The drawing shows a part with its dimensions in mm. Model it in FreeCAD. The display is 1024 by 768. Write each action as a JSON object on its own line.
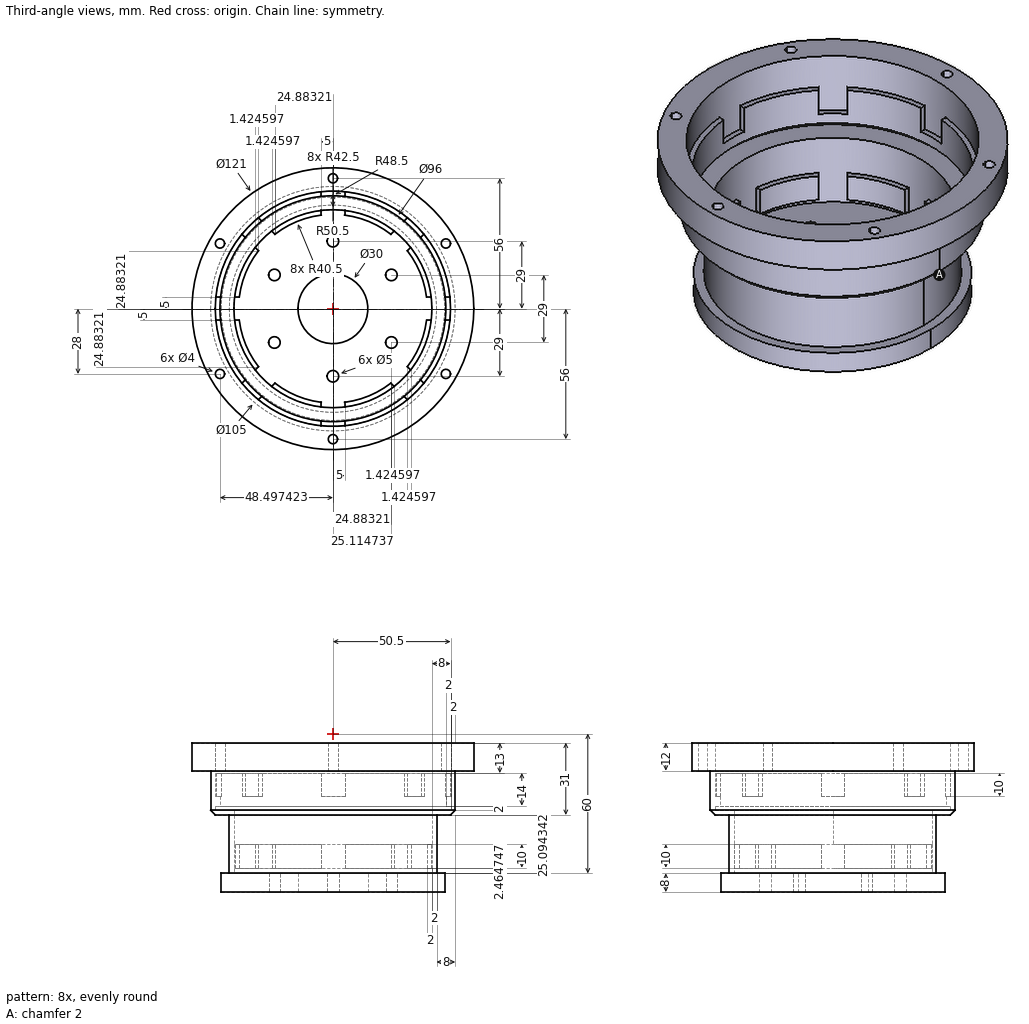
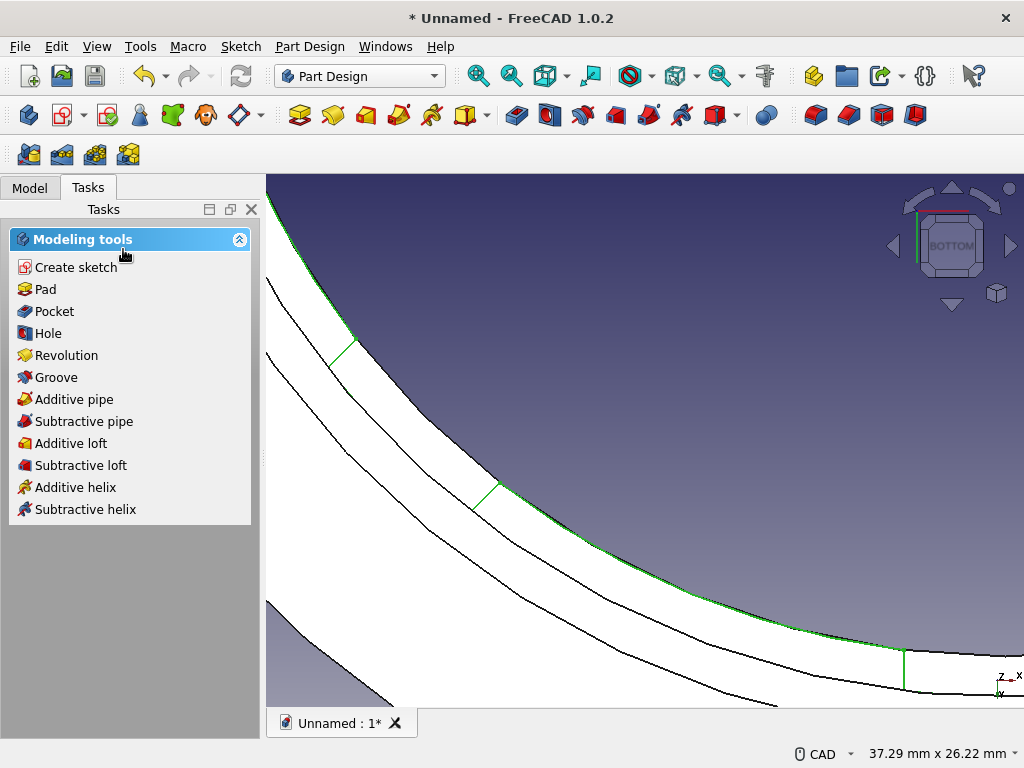
{"action": "left_click", "coordinate": [517, 116]}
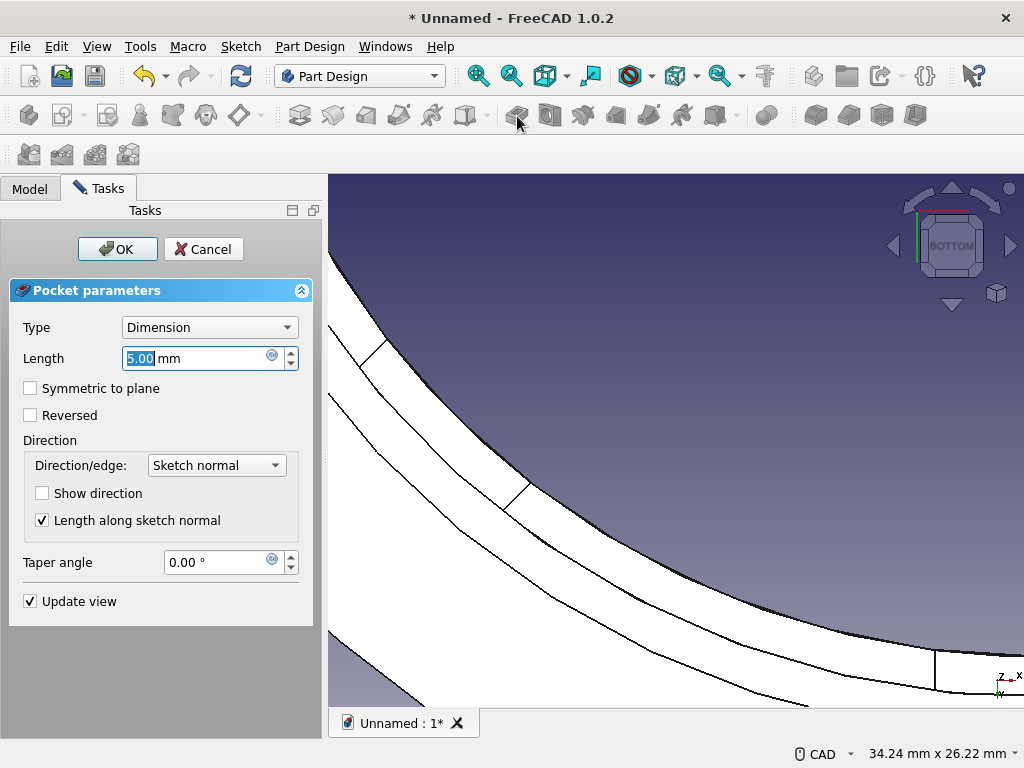
{"action": "type", "text": "10"}
{"action": "key", "text": "Tab"}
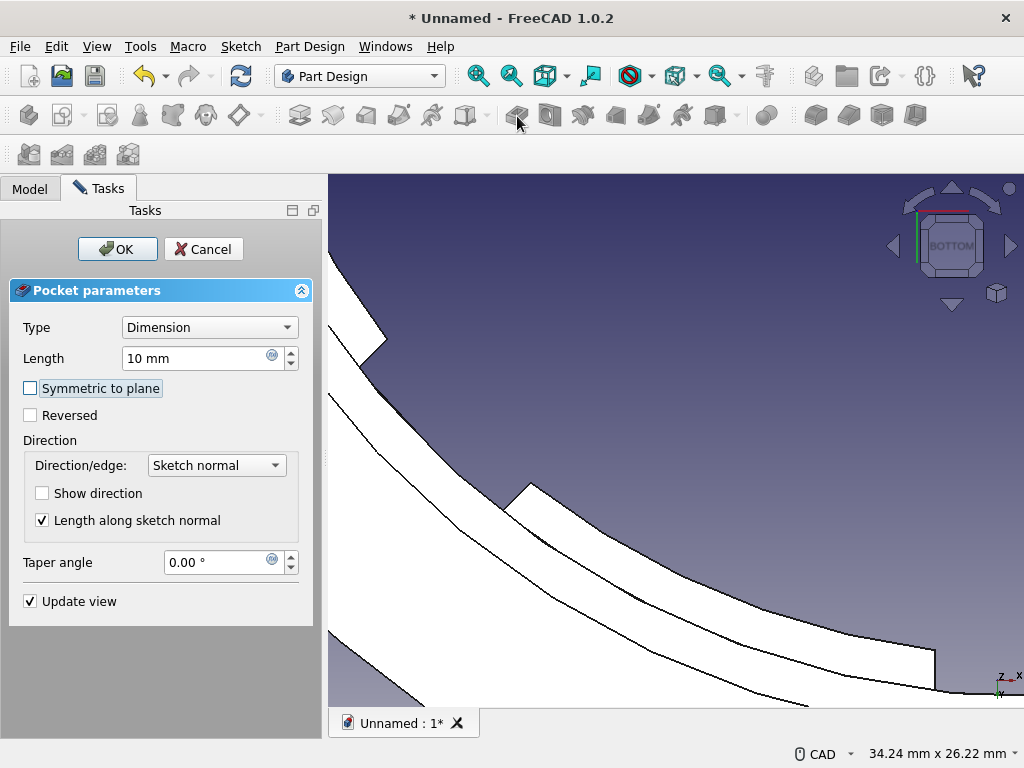
{"action": "left_click", "coordinate": [118, 249]}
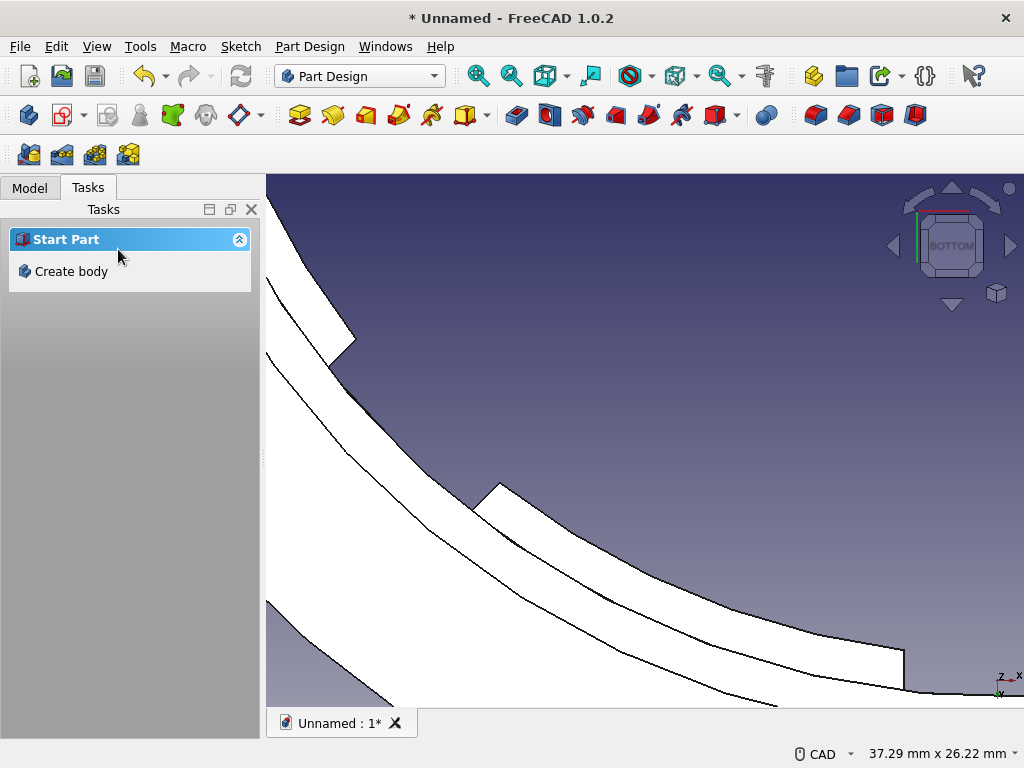
{"action": "left_click", "coordinate": [479, 76]}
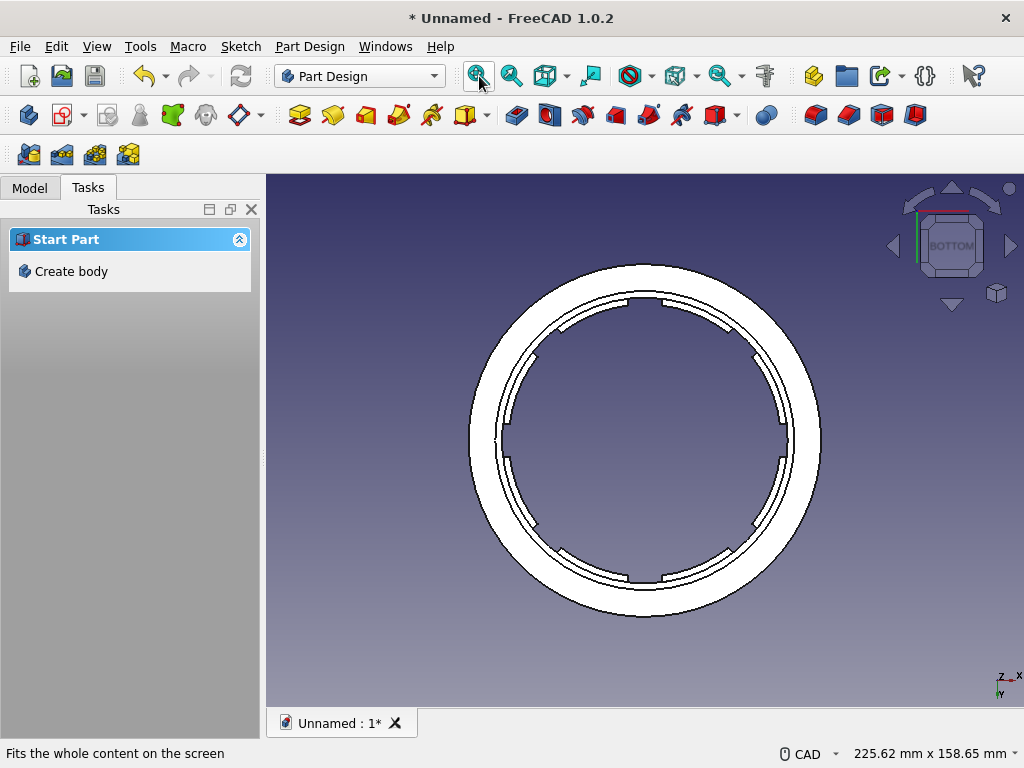
{"action": "left_click", "coordinate": [30, 188]}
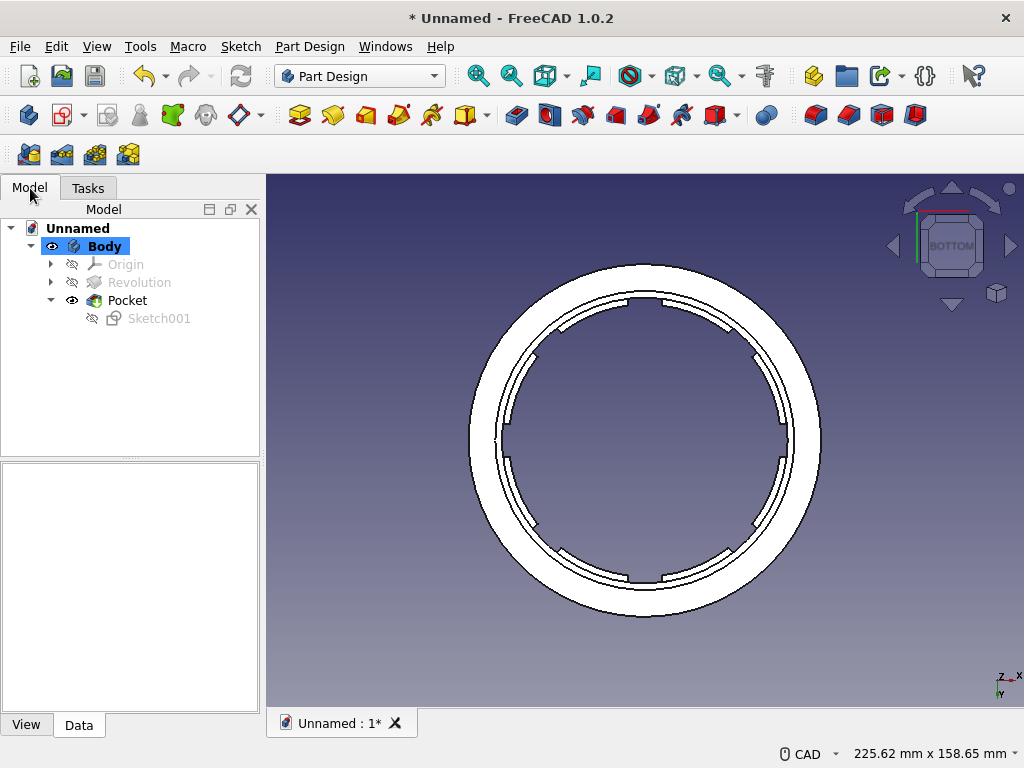
{"action": "left_click", "coordinate": [51, 264]}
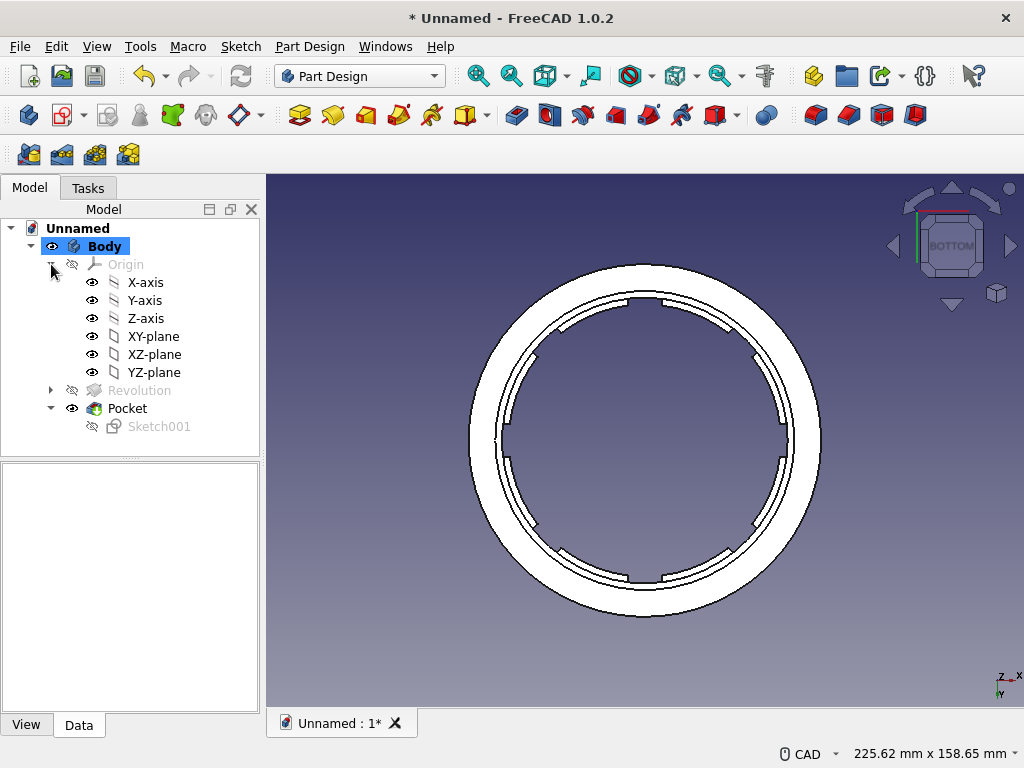
{"action": "left_click", "coordinate": [137, 336]}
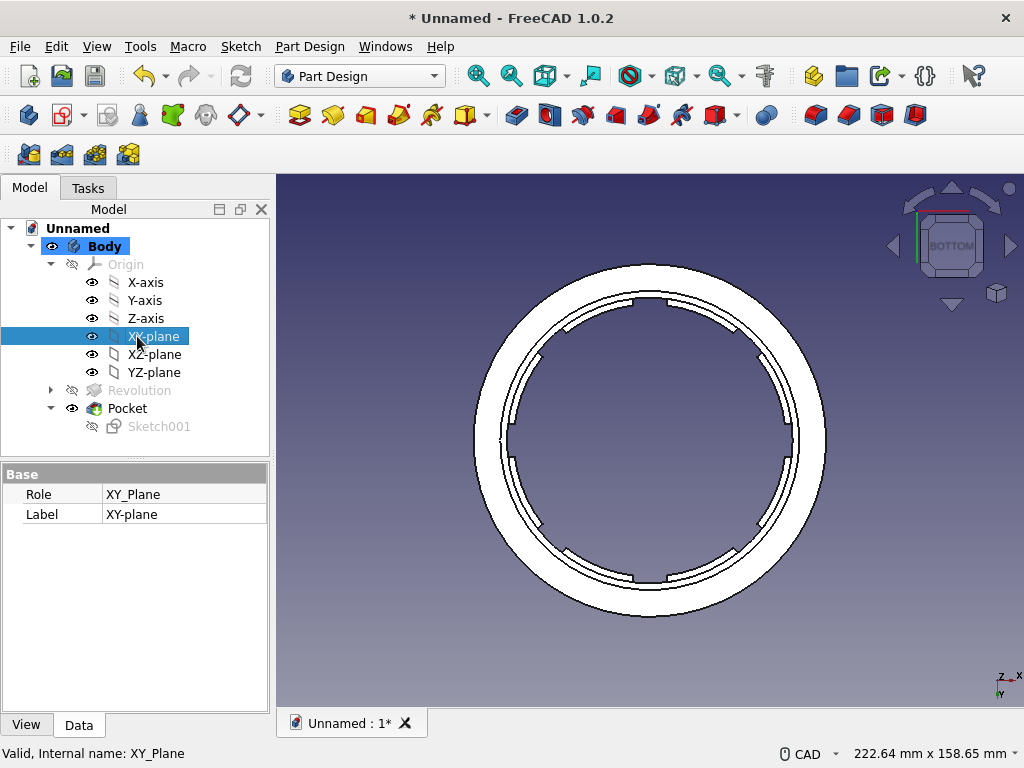
{"action": "left_click", "coordinate": [238, 116]}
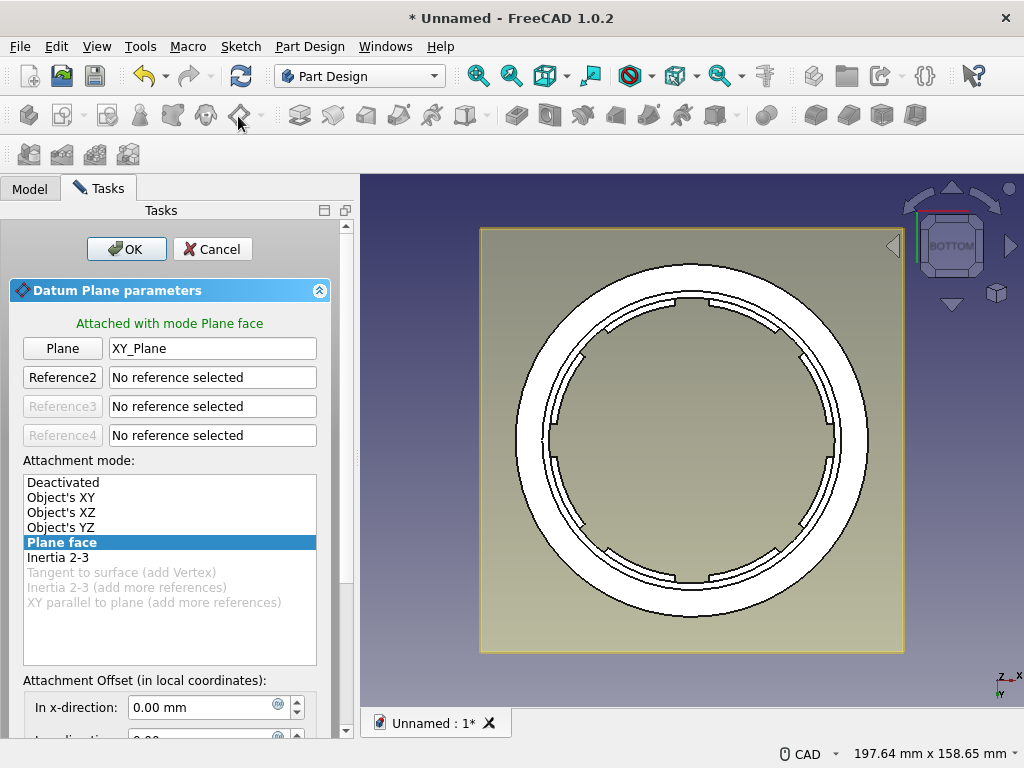
{"action": "scroll", "coordinate": [346, 479], "scroll_direction": "down", "scroll_amount": 2}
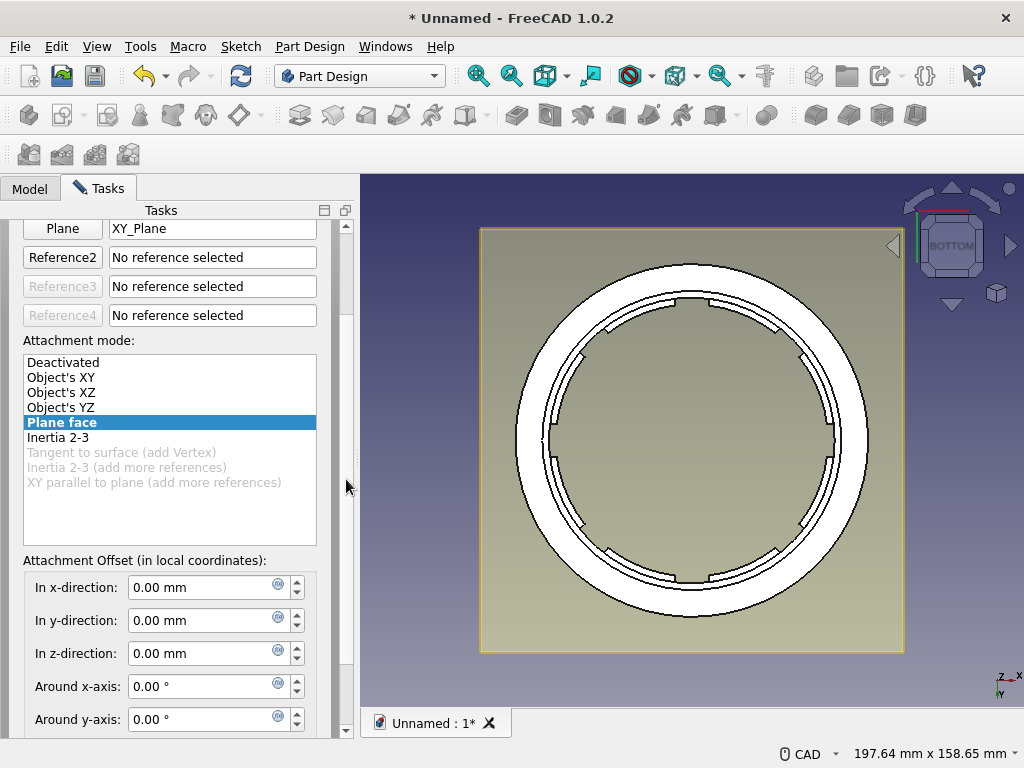
{"action": "triple_click", "coordinate": [210, 654]}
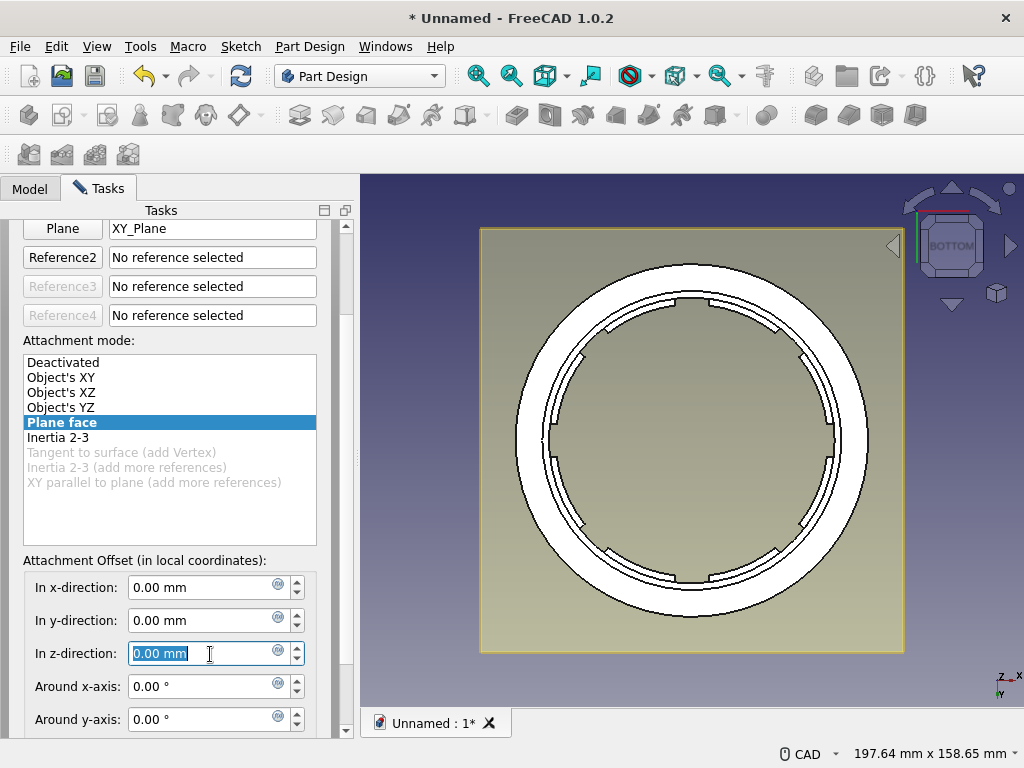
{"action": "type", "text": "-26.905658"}
{"action": "key", "text": "Tab"}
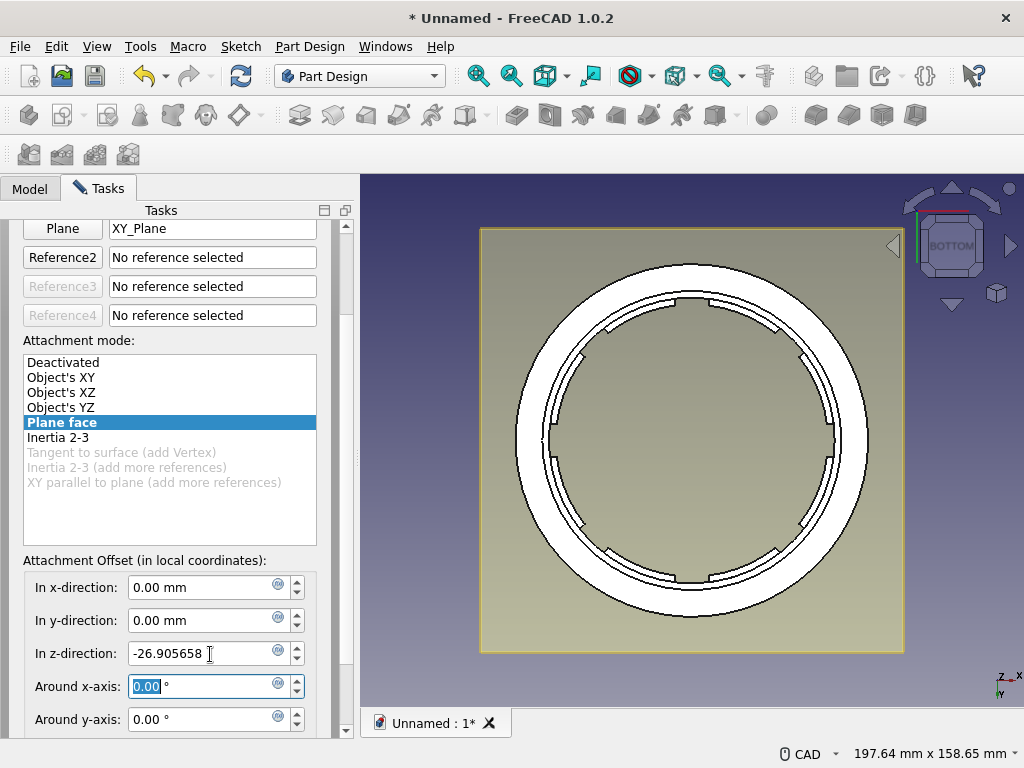
{"action": "scroll", "coordinate": [346, 479], "scroll_direction": "up", "scroll_amount": 3}